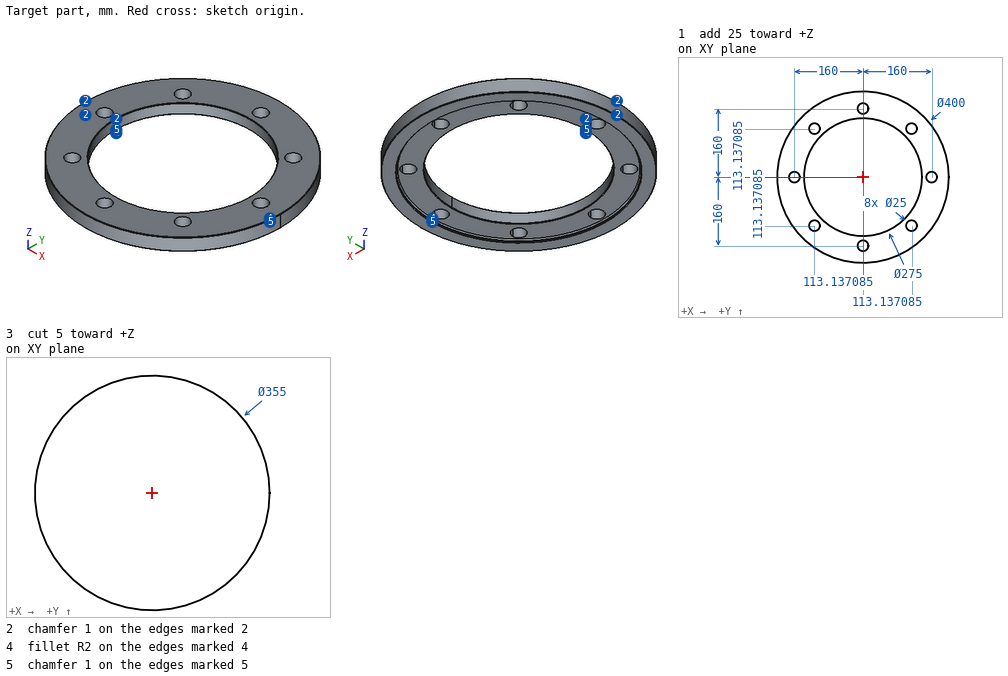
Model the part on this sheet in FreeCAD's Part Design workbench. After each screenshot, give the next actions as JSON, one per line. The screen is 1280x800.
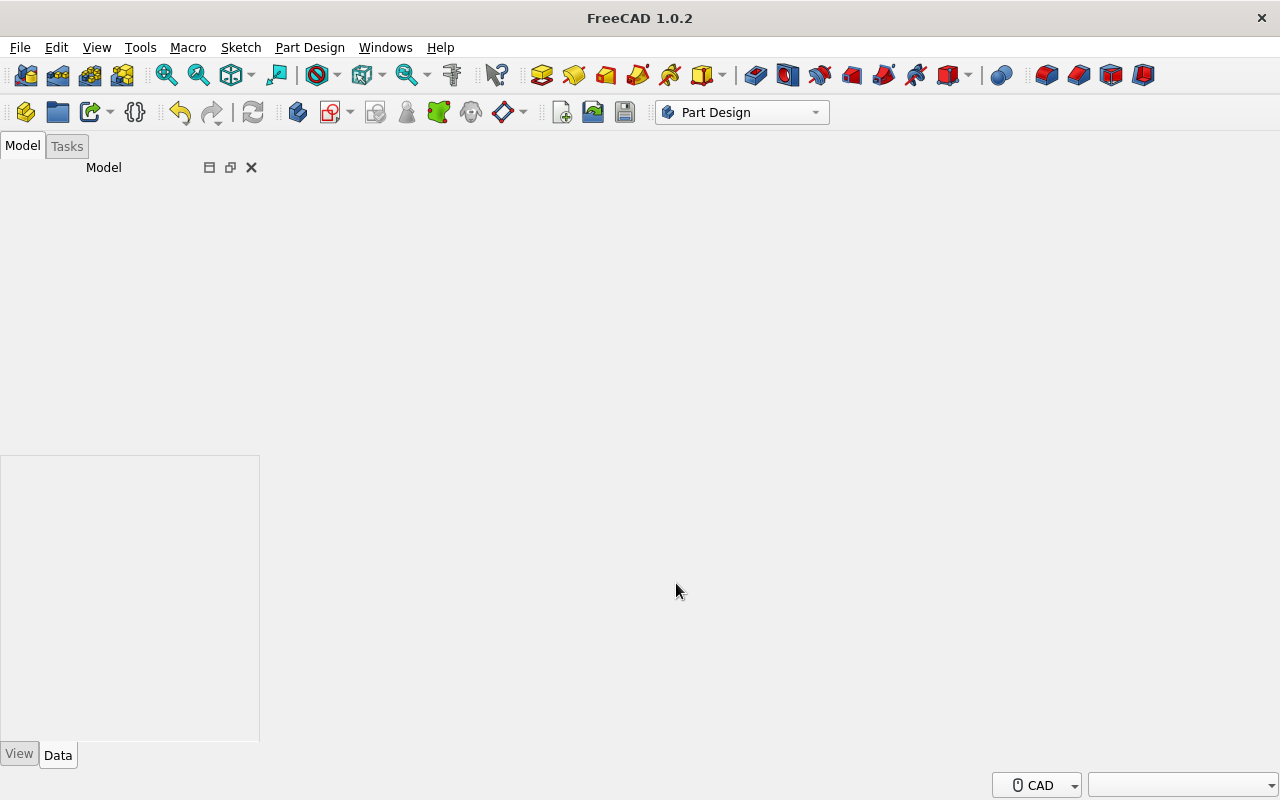
{"action": "left_click", "coordinate": [562, 112]}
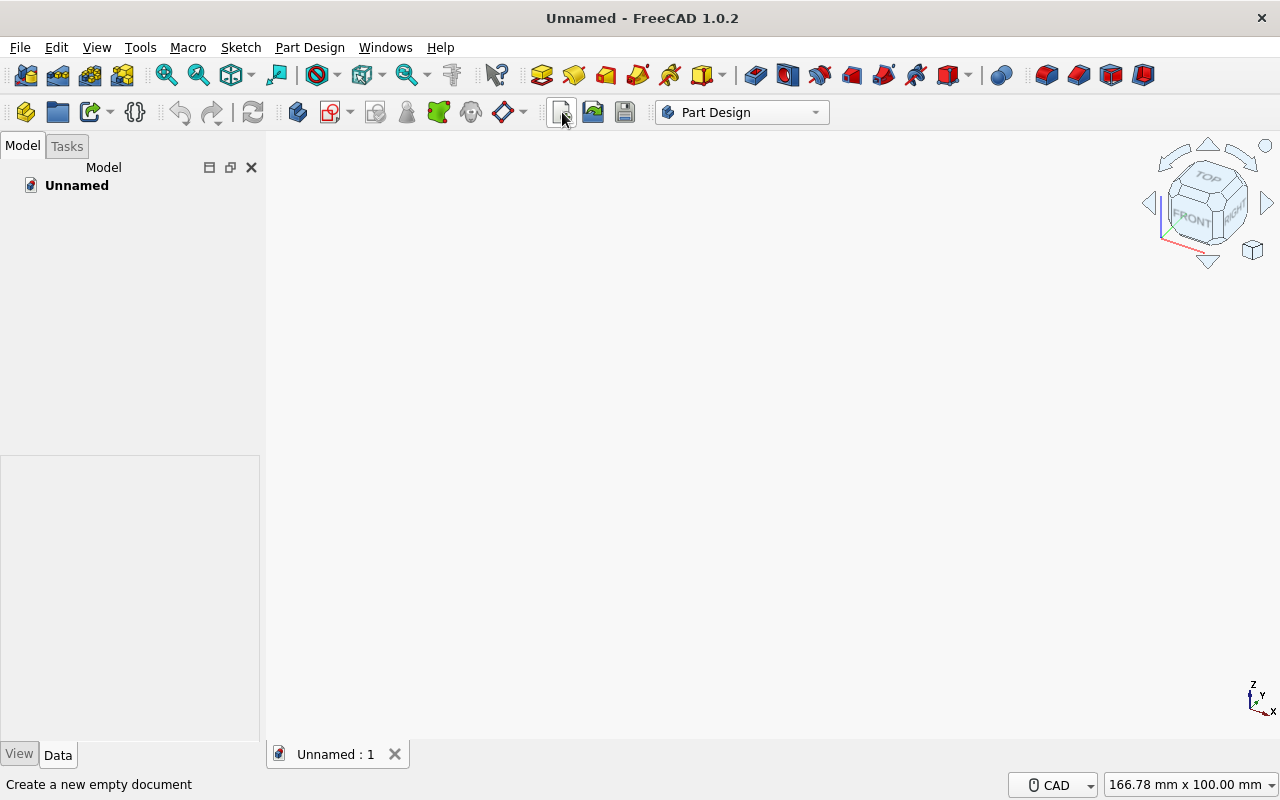
{"action": "left_click", "coordinate": [330, 112]}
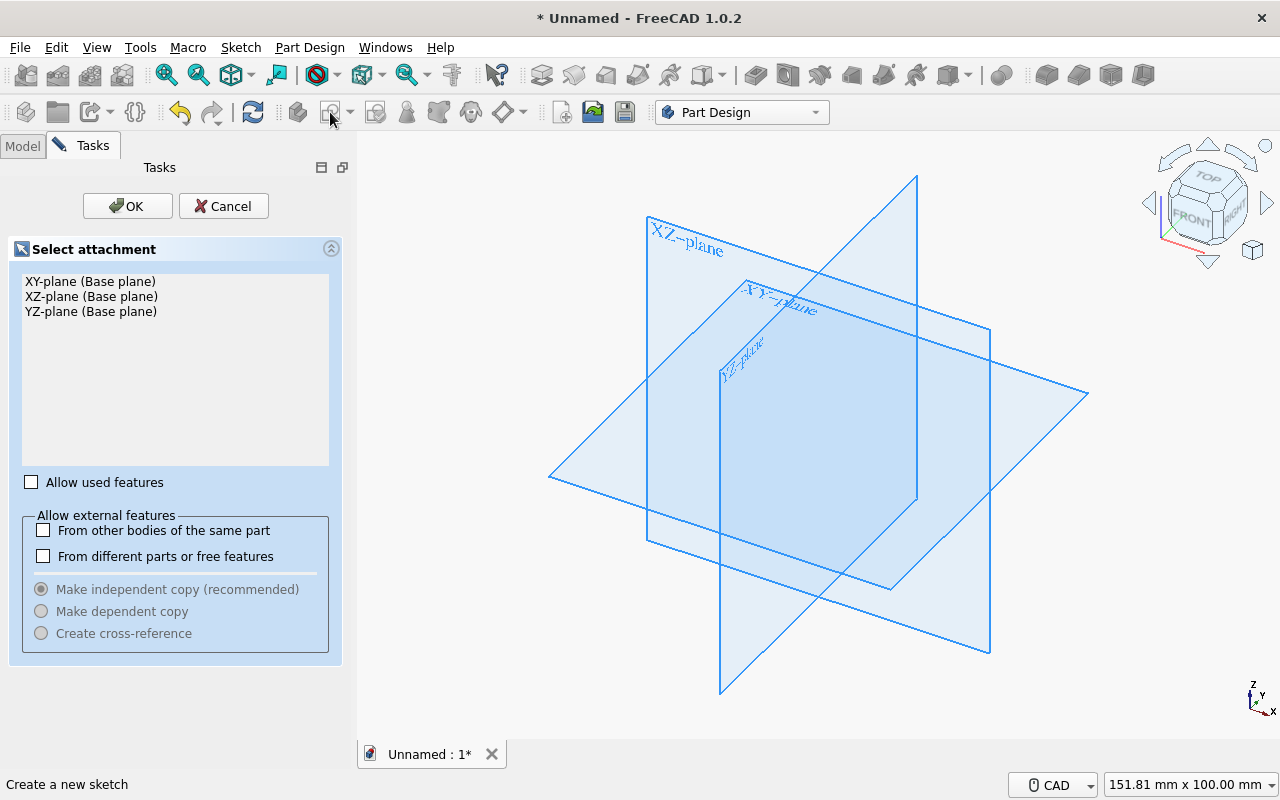
{"action": "left_click", "coordinate": [82, 282]}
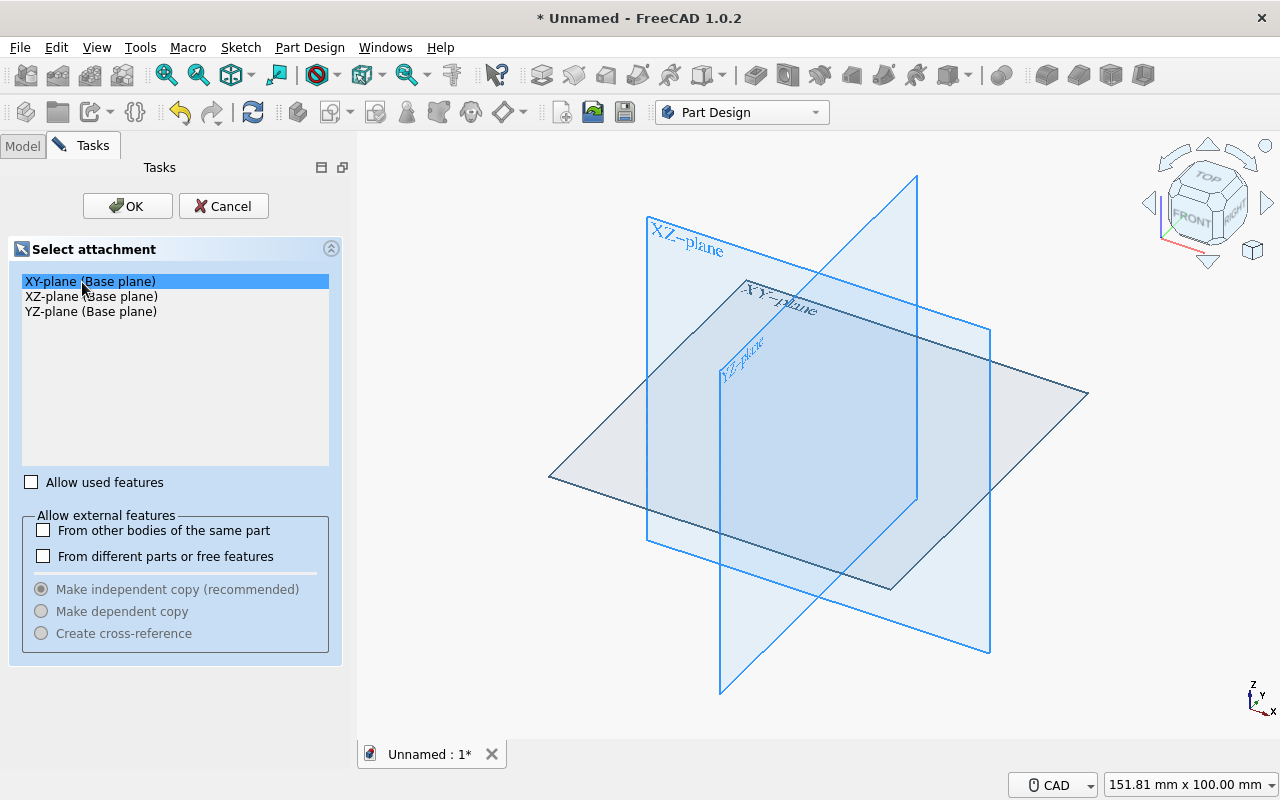
{"action": "left_click", "coordinate": [128, 206]}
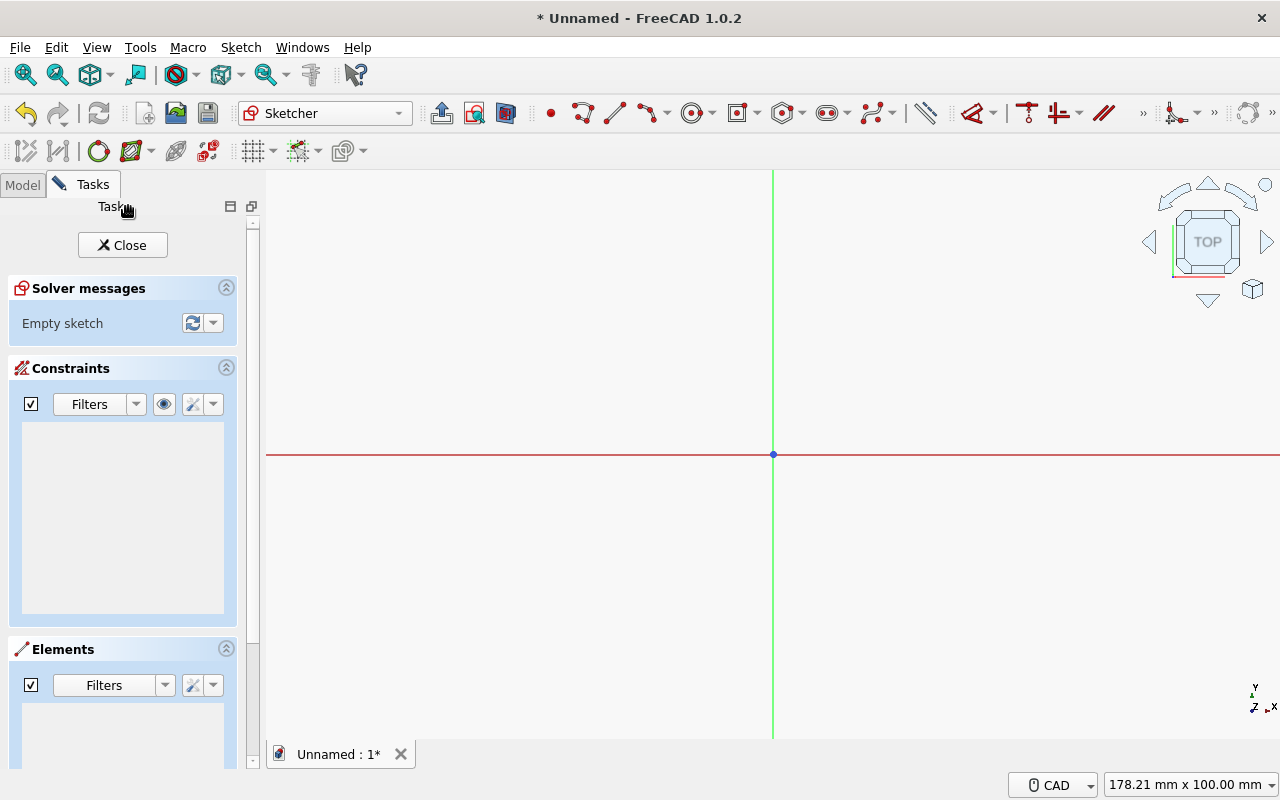
{"action": "scroll", "coordinate": [691, 454], "scroll_direction": "down", "scroll_amount": 9}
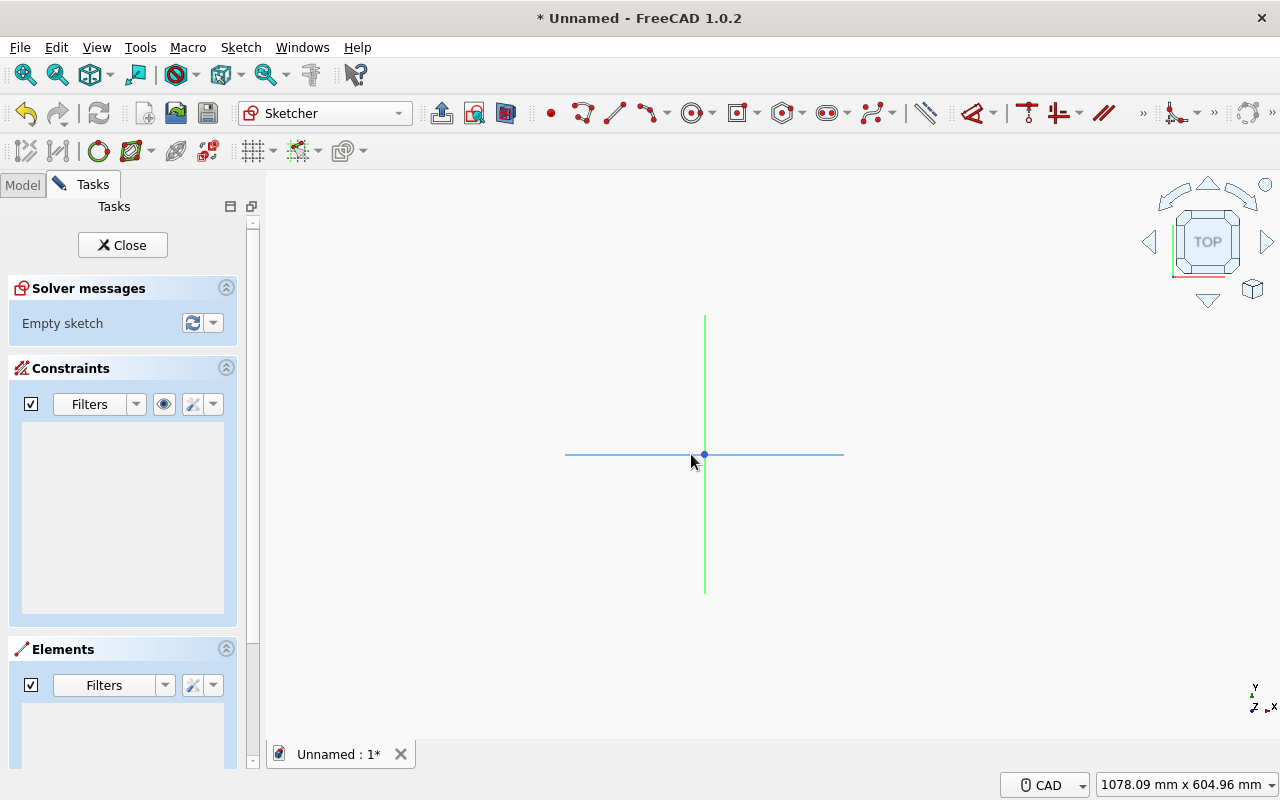
{"action": "left_click", "coordinate": [692, 114]}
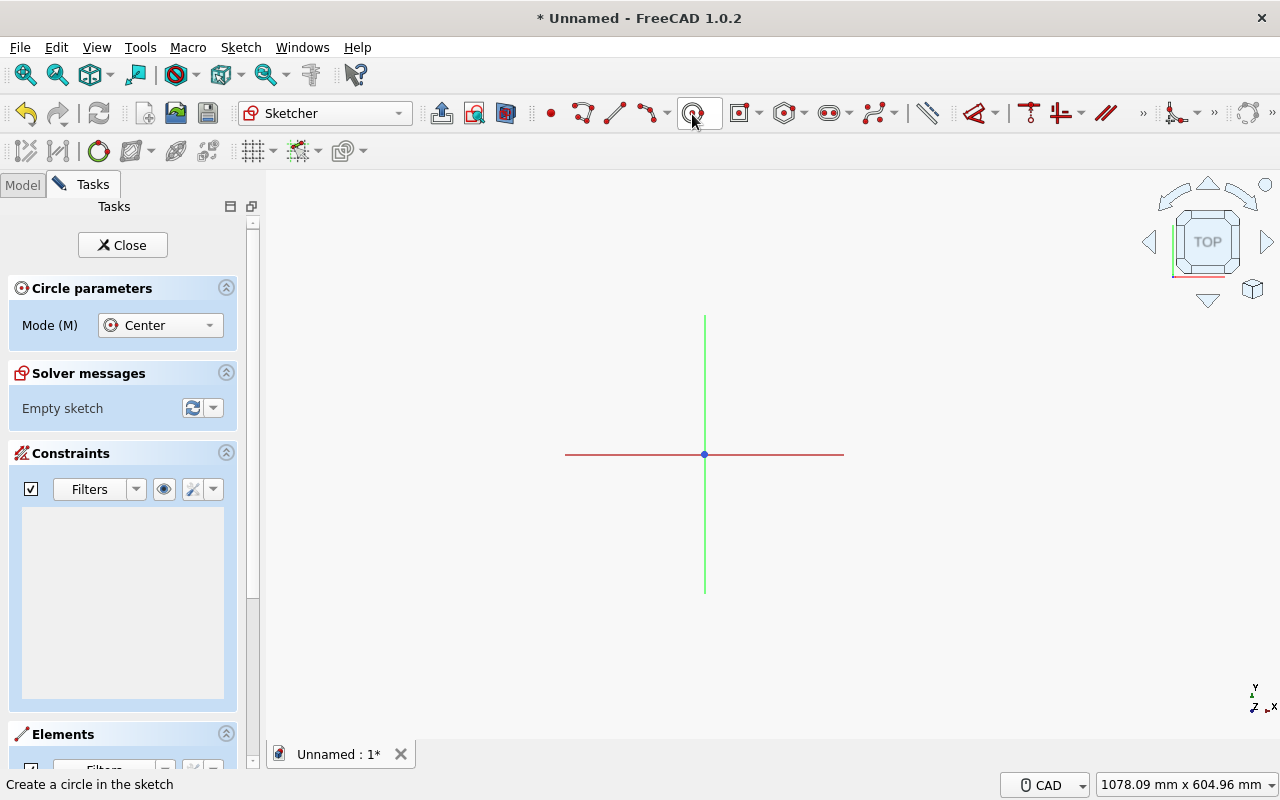
{"action": "left_click", "coordinate": [705, 454]}
{"action": "left_click", "coordinate": [838, 321]}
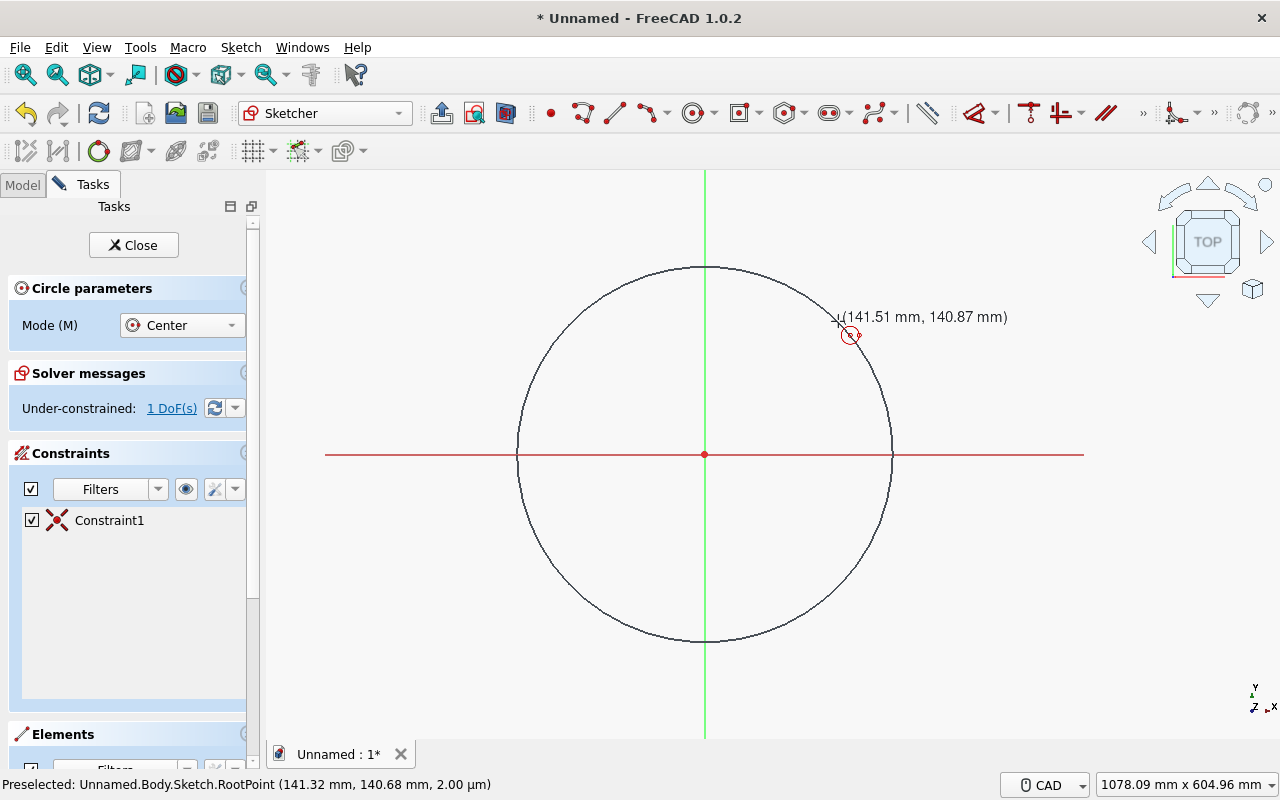
{"action": "scroll", "coordinate": [598, 561], "scroll_direction": "up", "scroll_amount": 4}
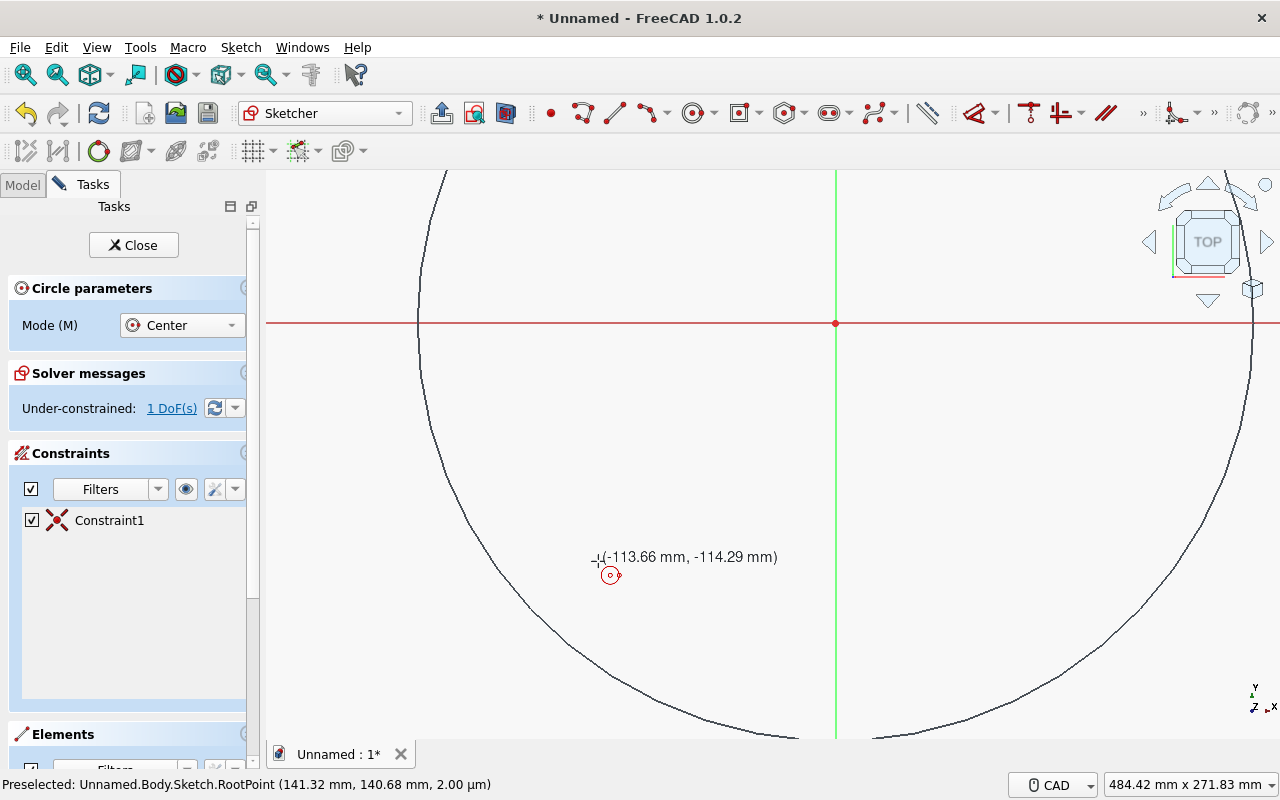
{"action": "left_click", "coordinate": [599, 560]}
{"action": "left_click", "coordinate": [617, 541]}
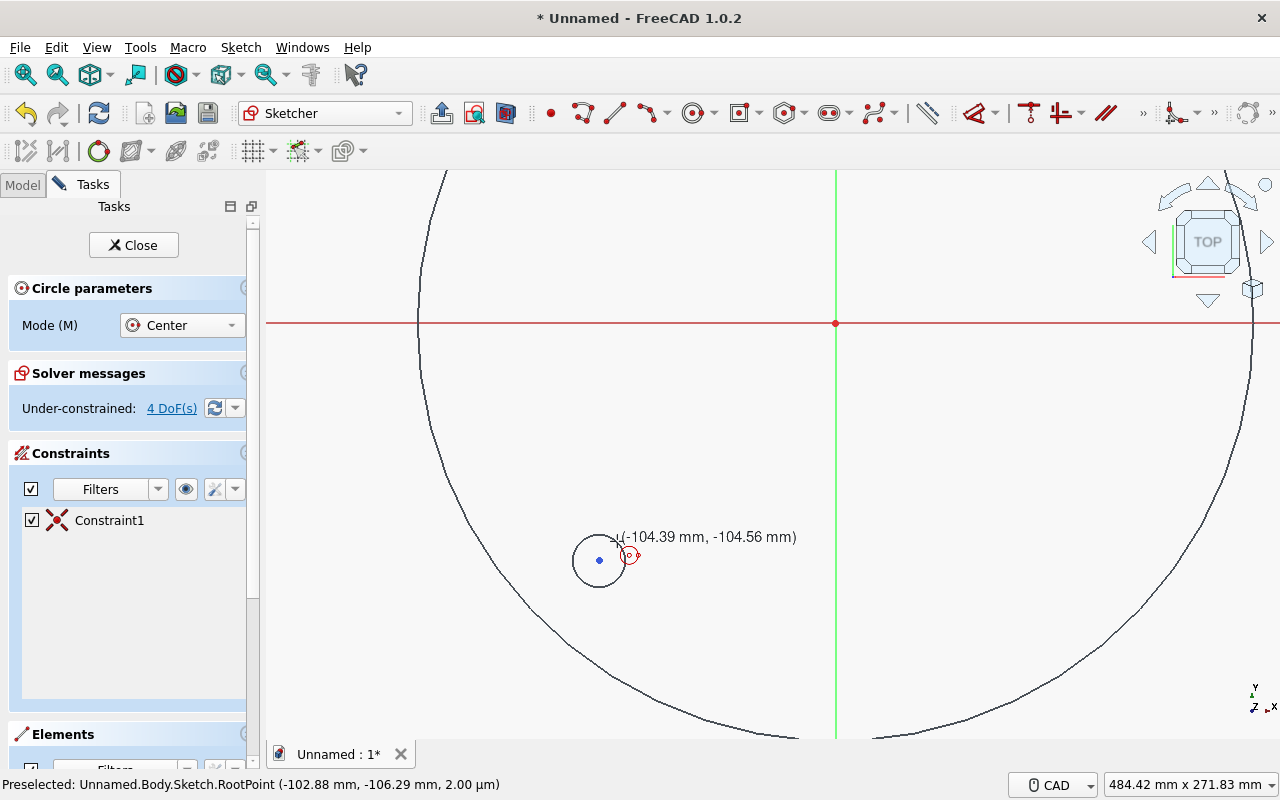
{"action": "left_click", "coordinate": [836, 658]}
{"action": "left_click", "coordinate": [854, 640]}